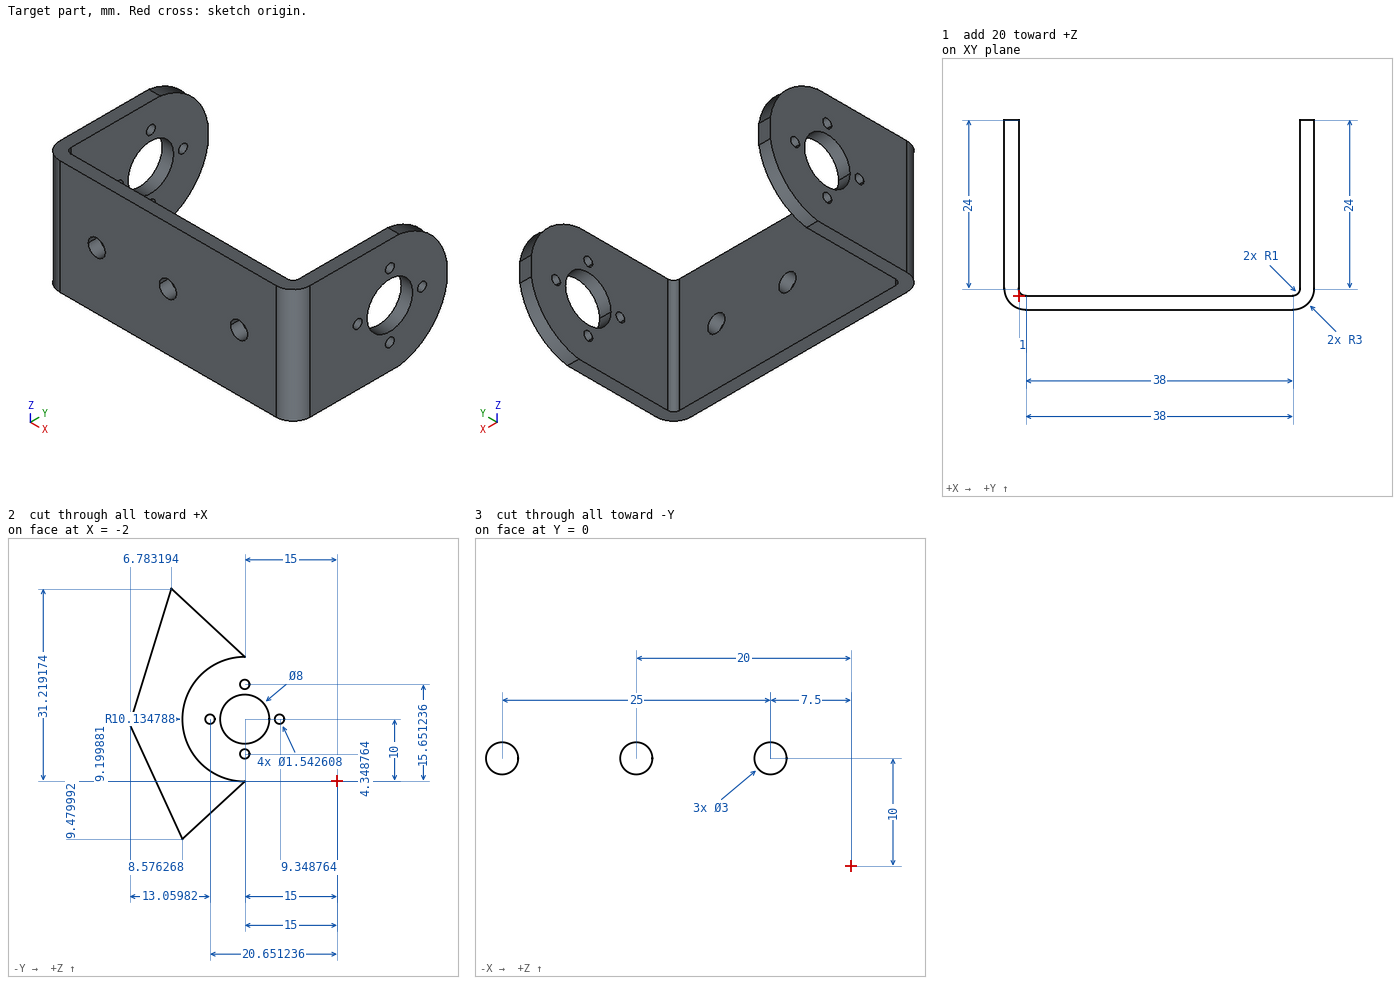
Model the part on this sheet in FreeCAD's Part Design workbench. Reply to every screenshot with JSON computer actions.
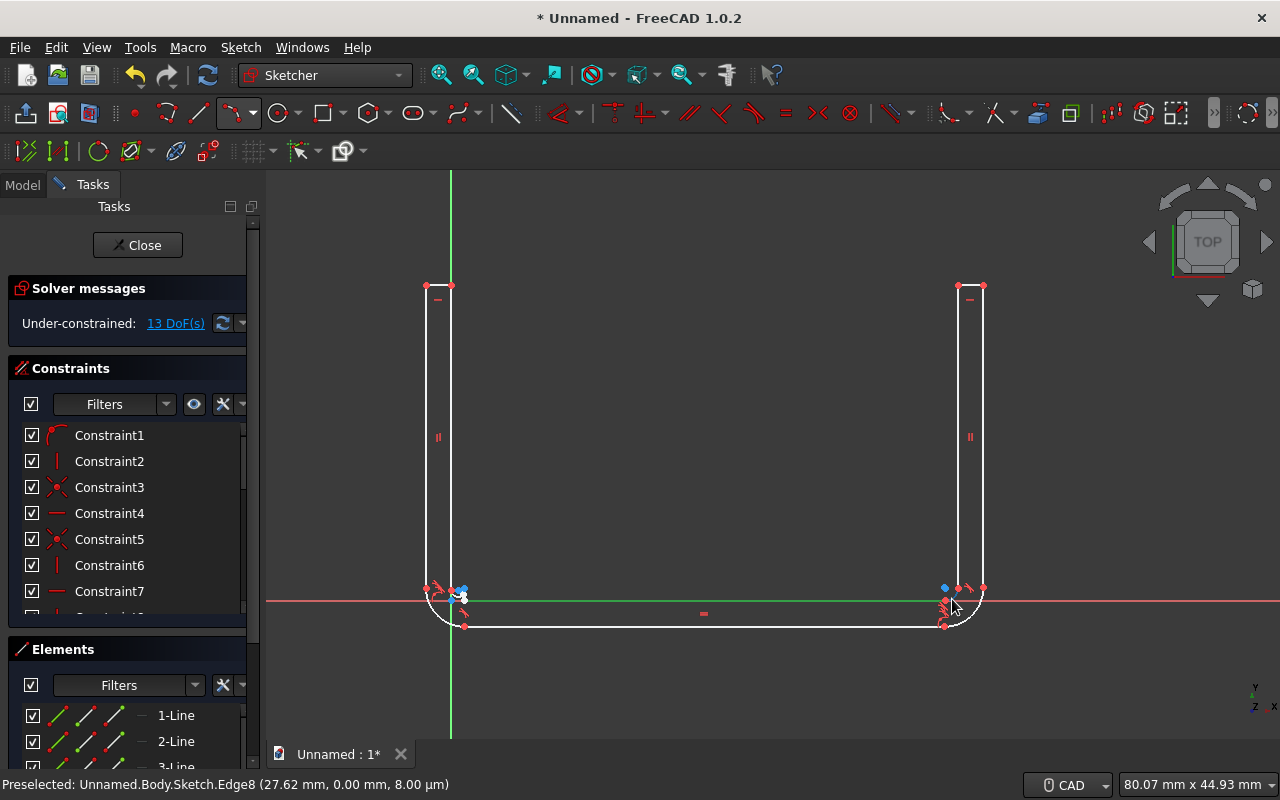
{"action": "scroll", "coordinate": [460, 597], "scroll_direction": "up", "scroll_amount": 7}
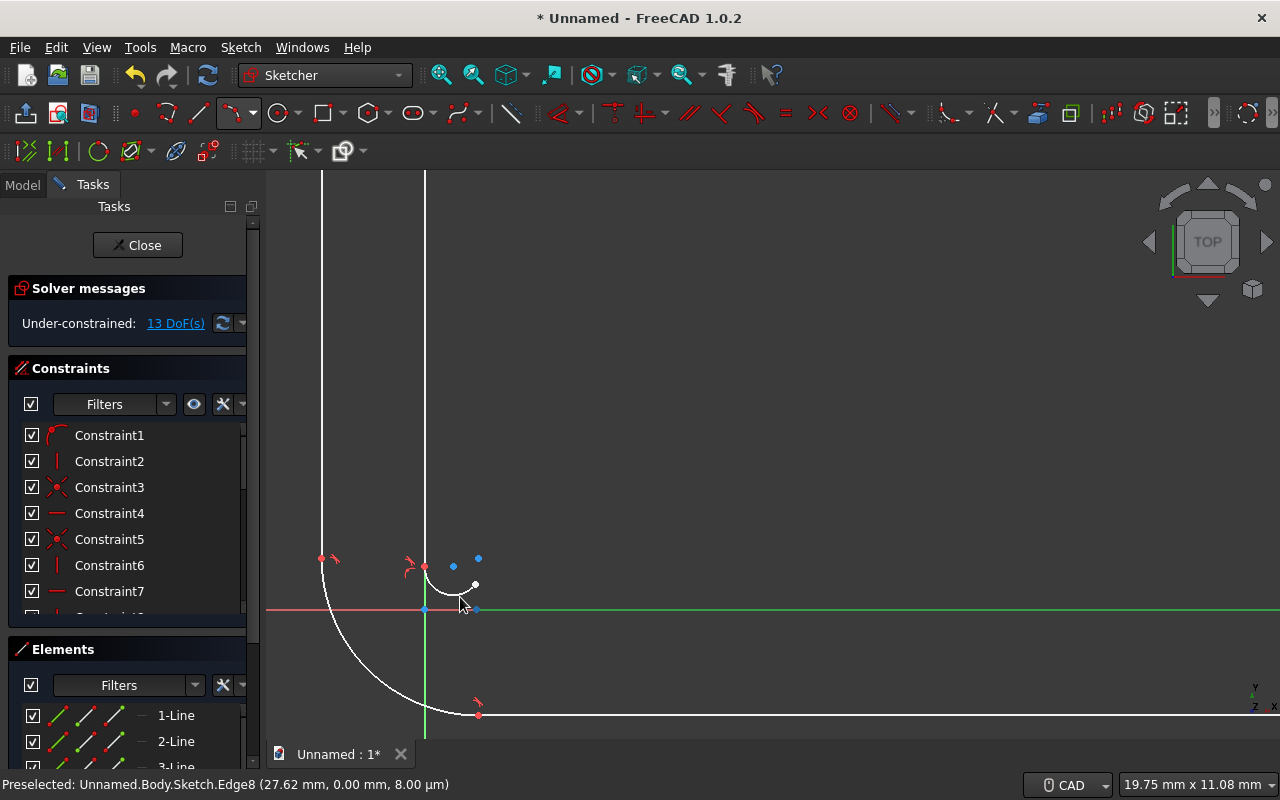
{"action": "left_click", "coordinate": [458, 595]}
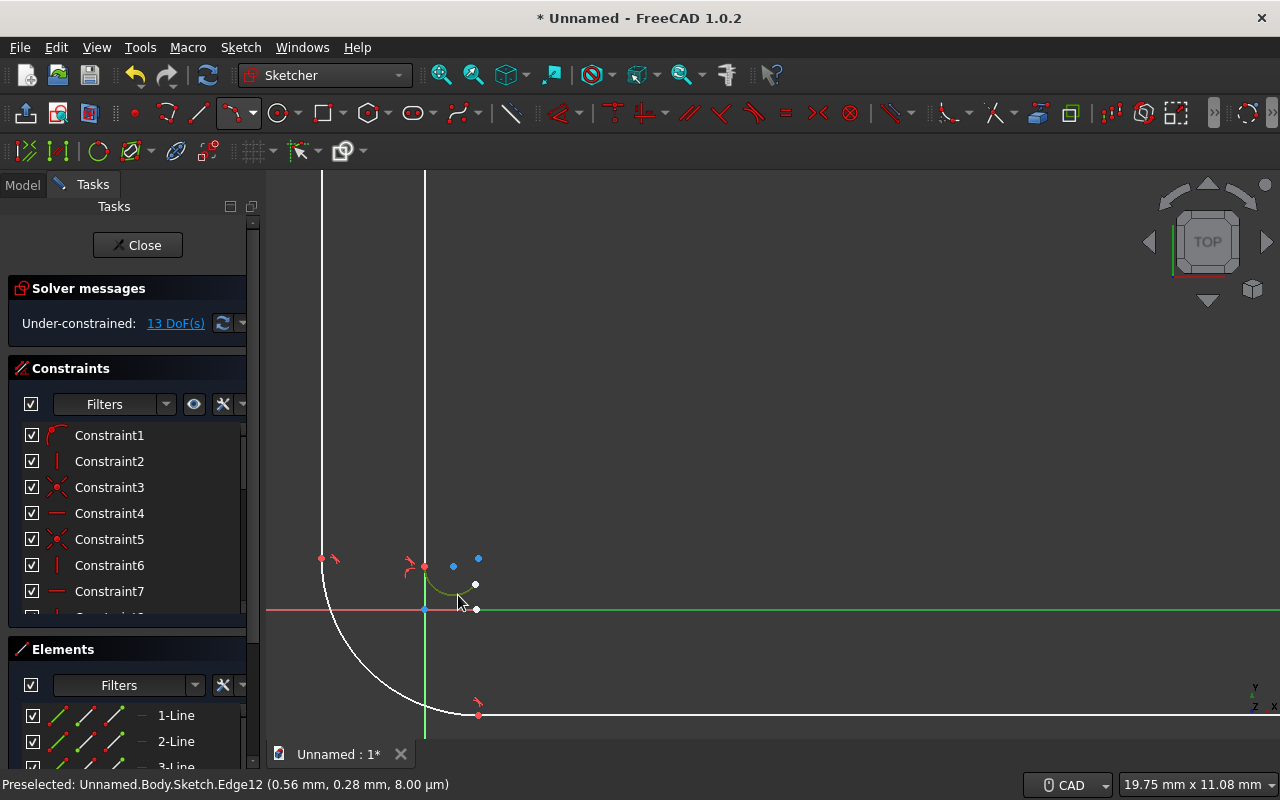
{"action": "left_click", "coordinate": [754, 114]}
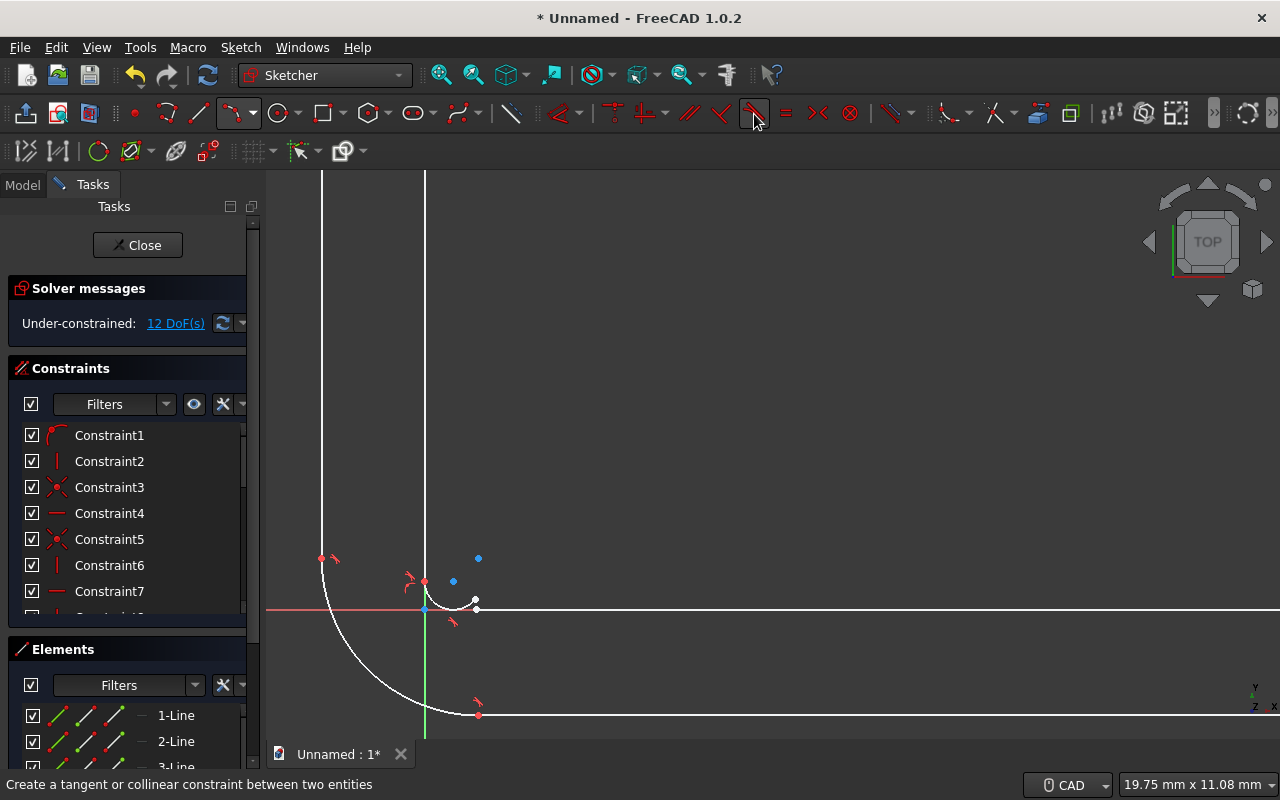
{"action": "scroll", "coordinate": [460, 597], "scroll_direction": "down", "scroll_amount": 7}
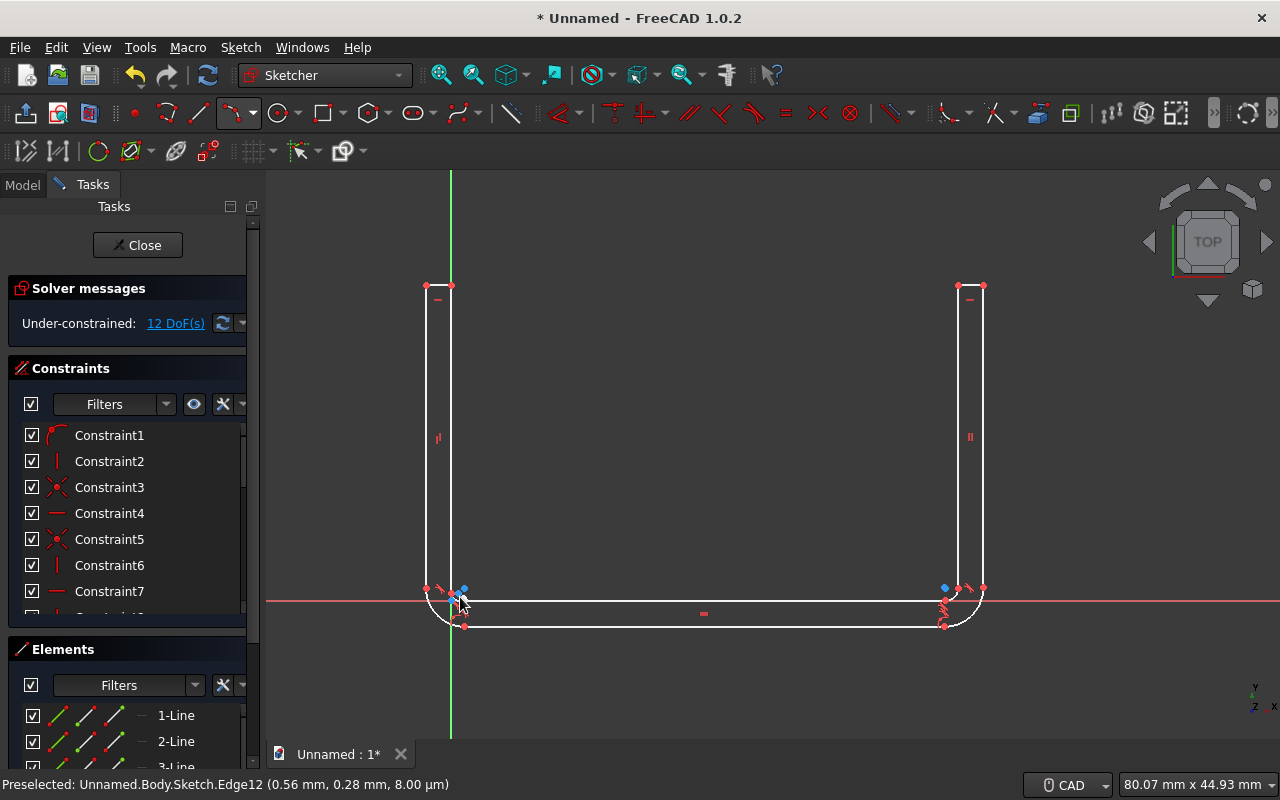
{"action": "left_click", "coordinate": [962, 623]}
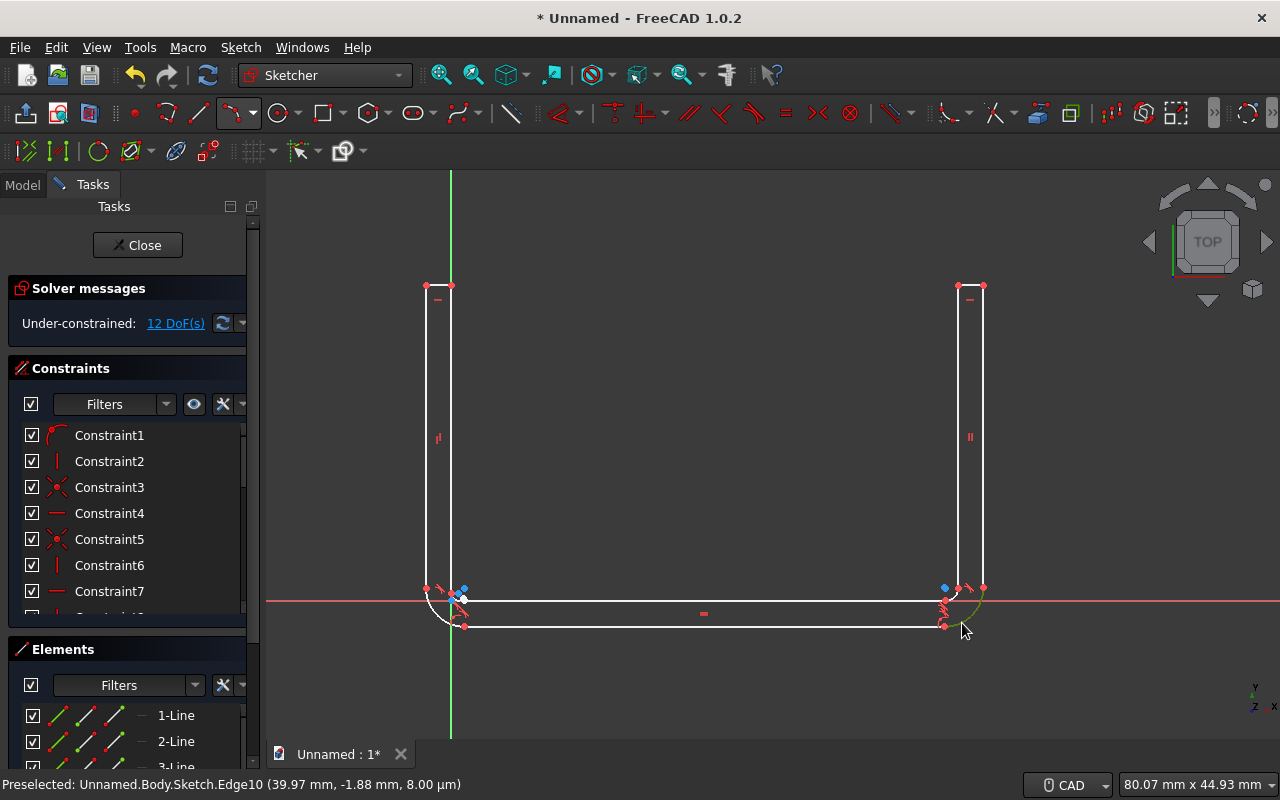
{"action": "scroll", "coordinate": [954, 597], "scroll_direction": "up", "scroll_amount": 2}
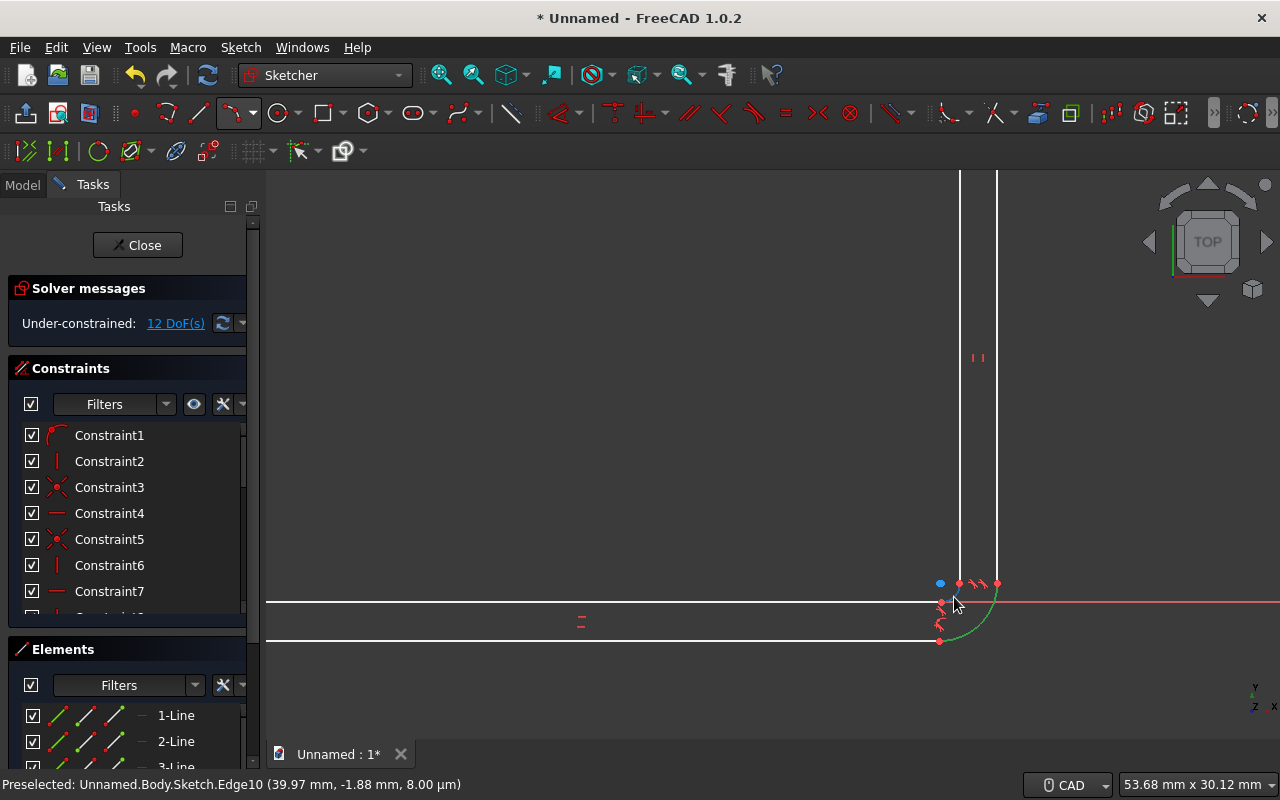
{"action": "left_click", "coordinate": [954, 597]}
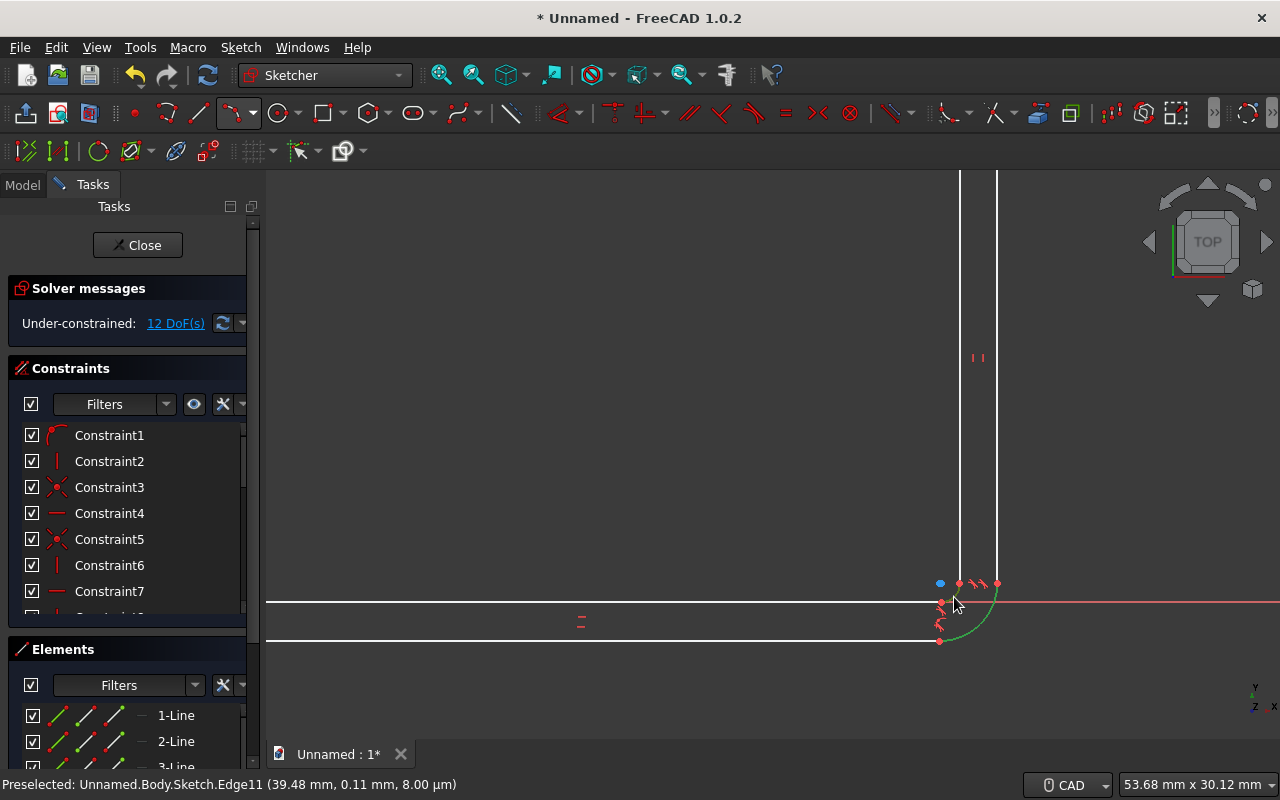
{"action": "left_click", "coordinate": [614, 114]}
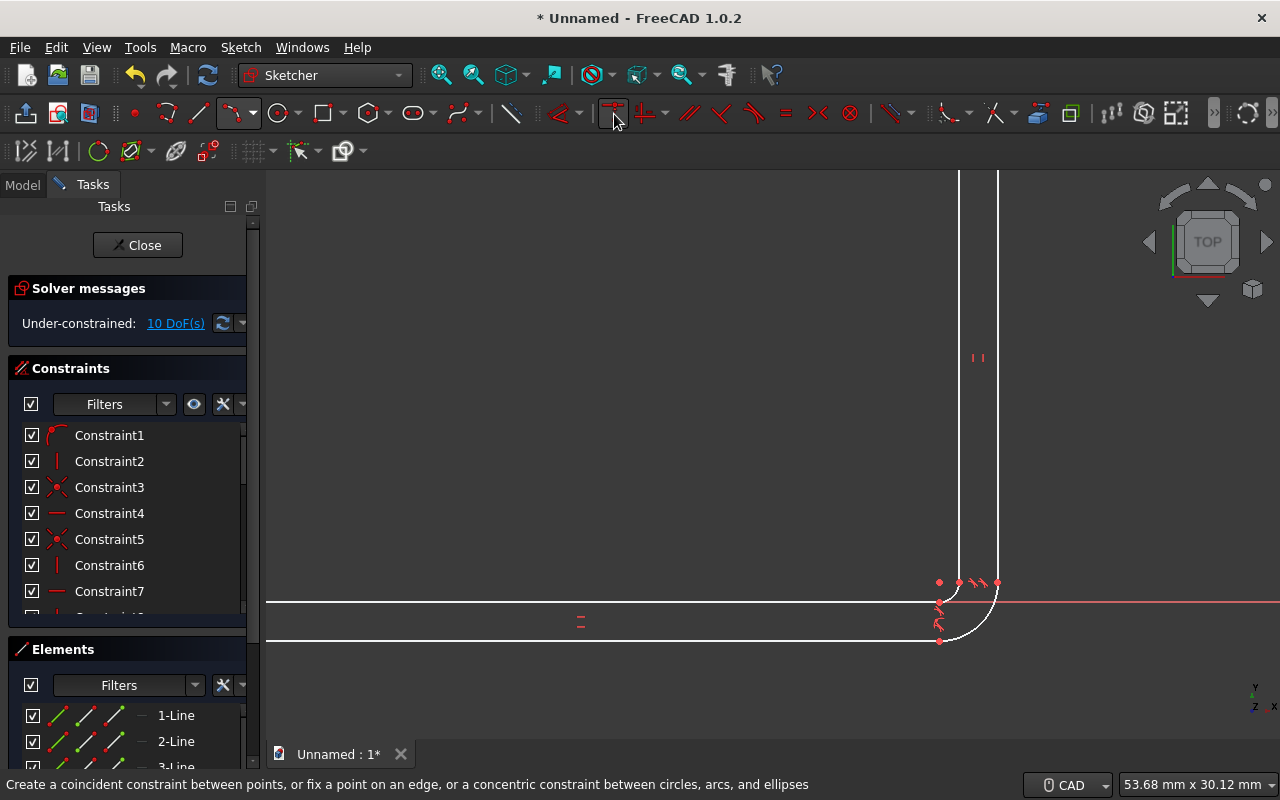
{"action": "scroll", "coordinate": [954, 596], "scroll_direction": "down", "scroll_amount": 2}